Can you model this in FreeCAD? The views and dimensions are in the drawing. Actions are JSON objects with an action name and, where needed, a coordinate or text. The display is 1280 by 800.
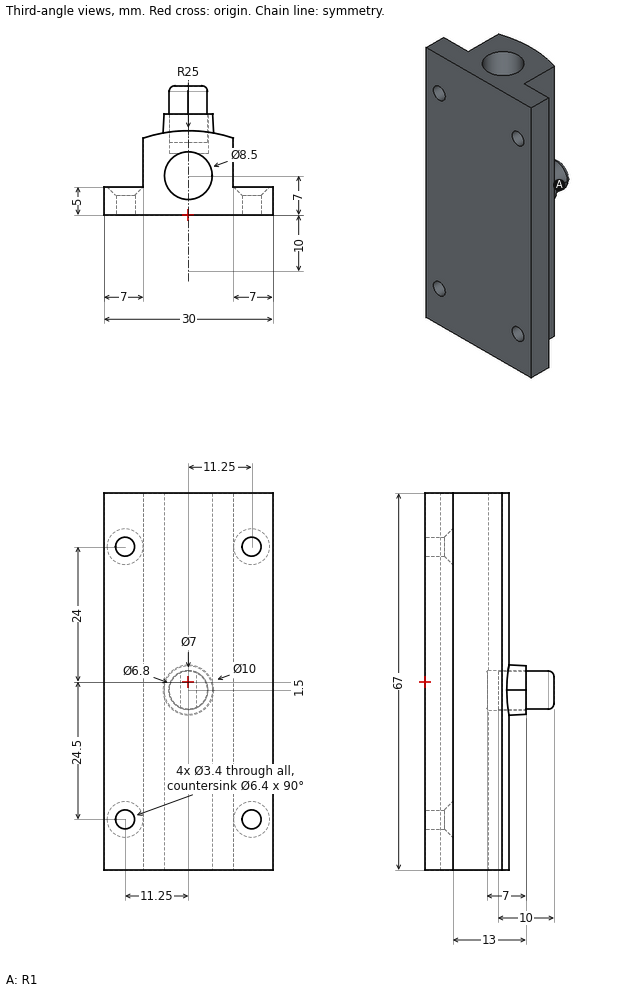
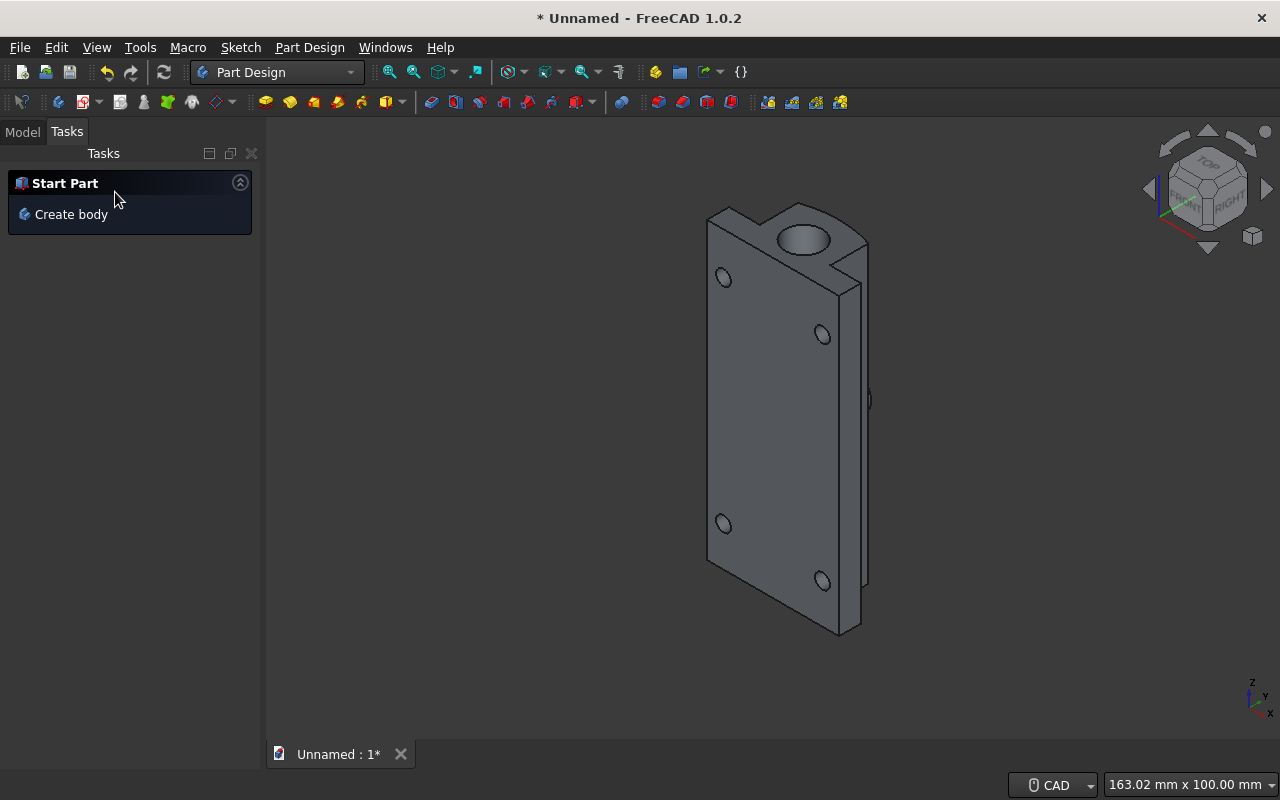
{"action": "left_click", "coordinate": [60, 102]}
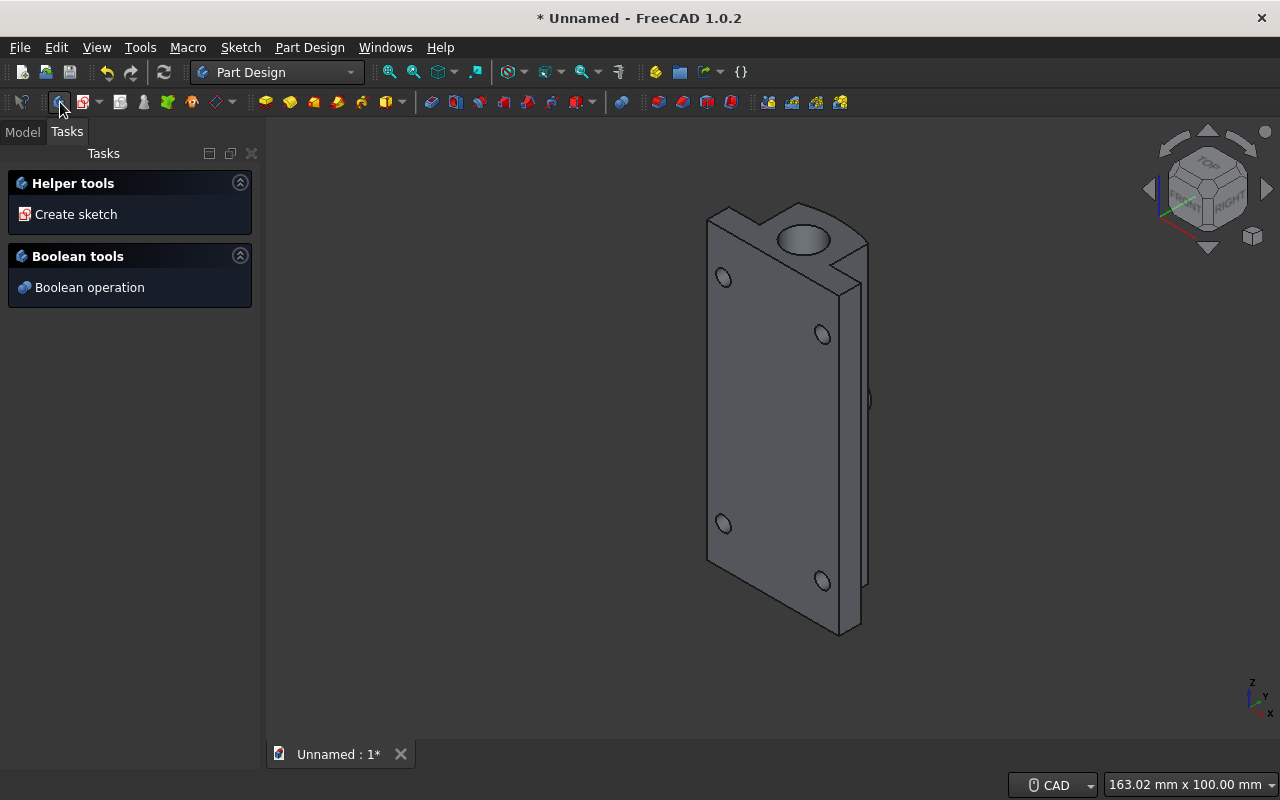
{"action": "left_click", "coordinate": [23, 131]}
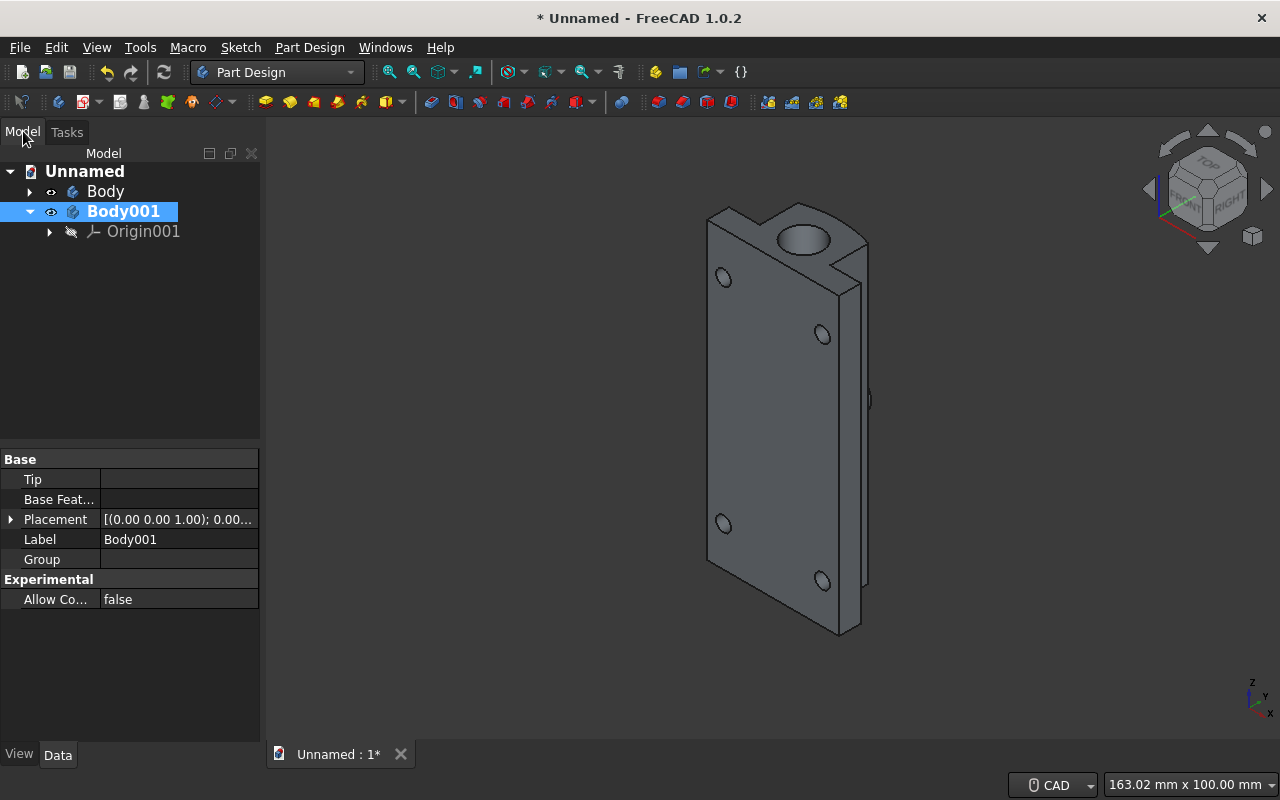
{"action": "left_click", "coordinate": [50, 232]}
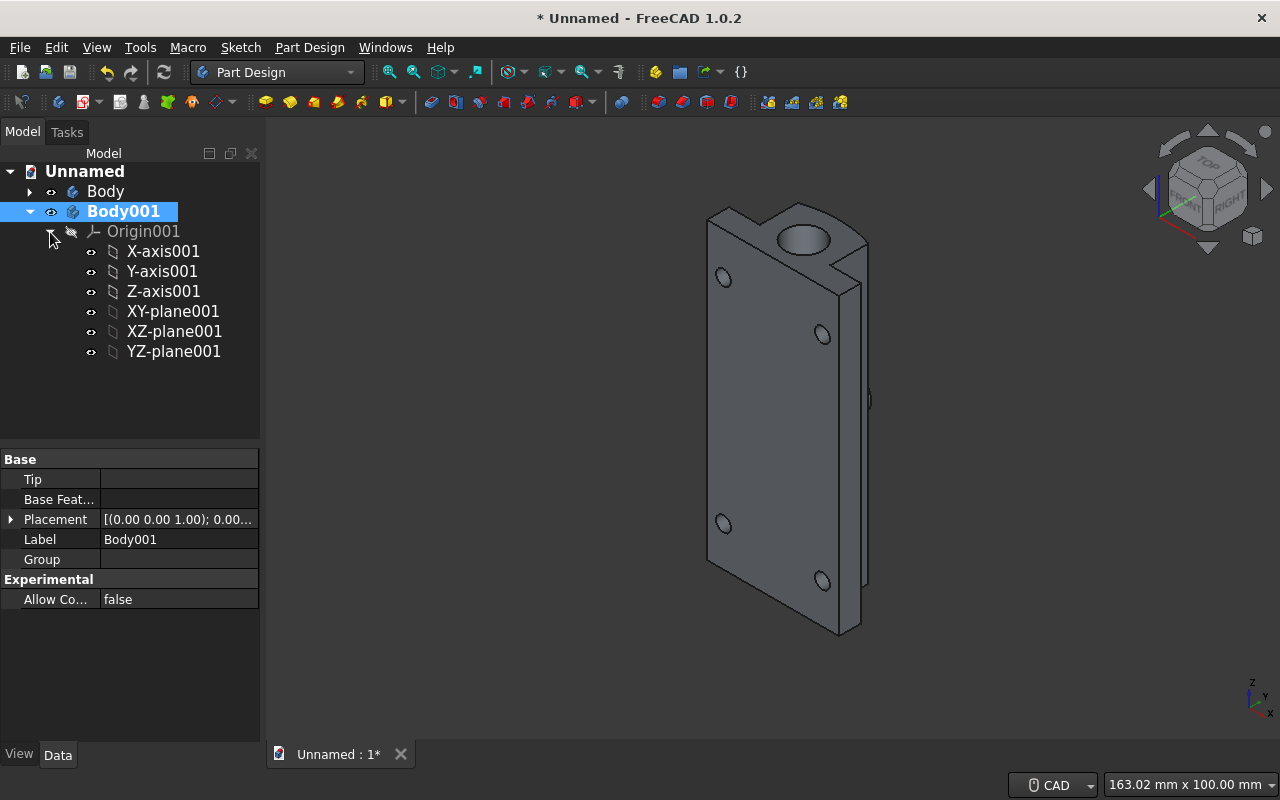
{"action": "left_click", "coordinate": [136, 332]}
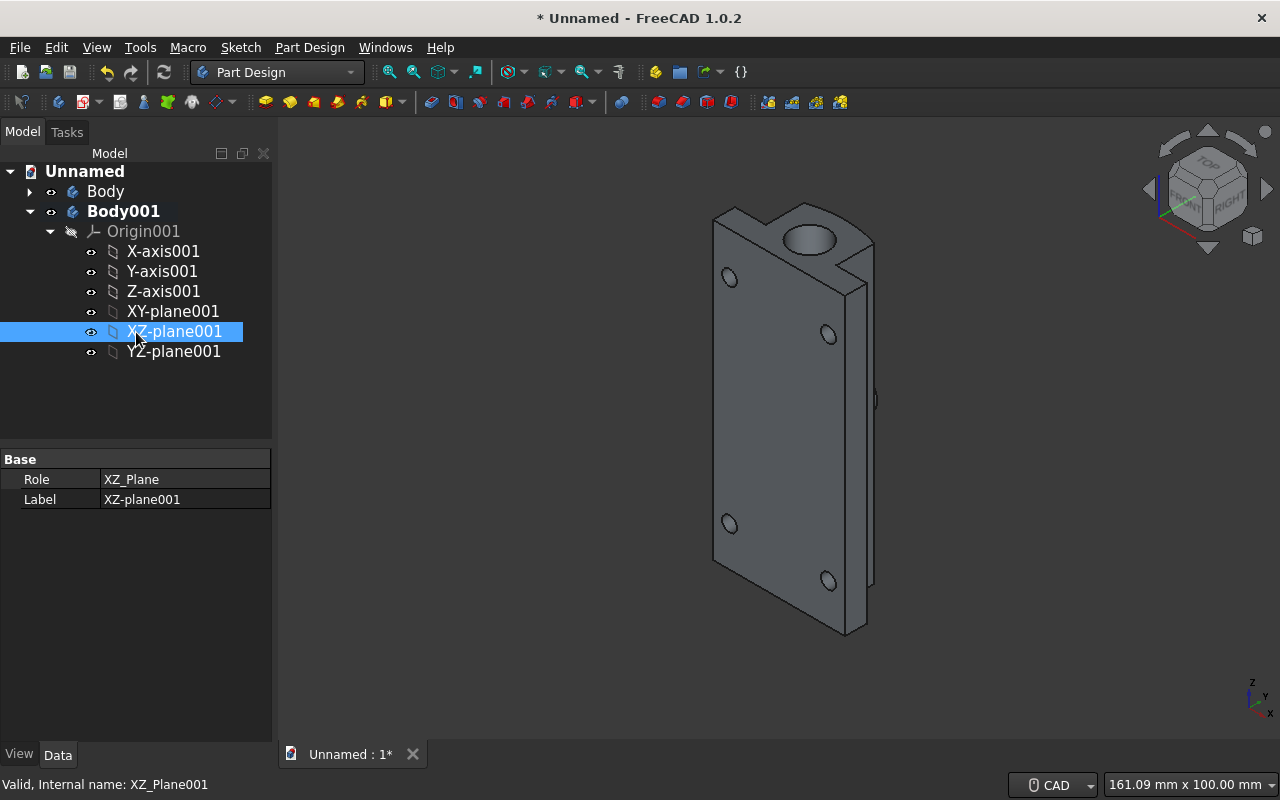
{"action": "left_click", "coordinate": [216, 102]}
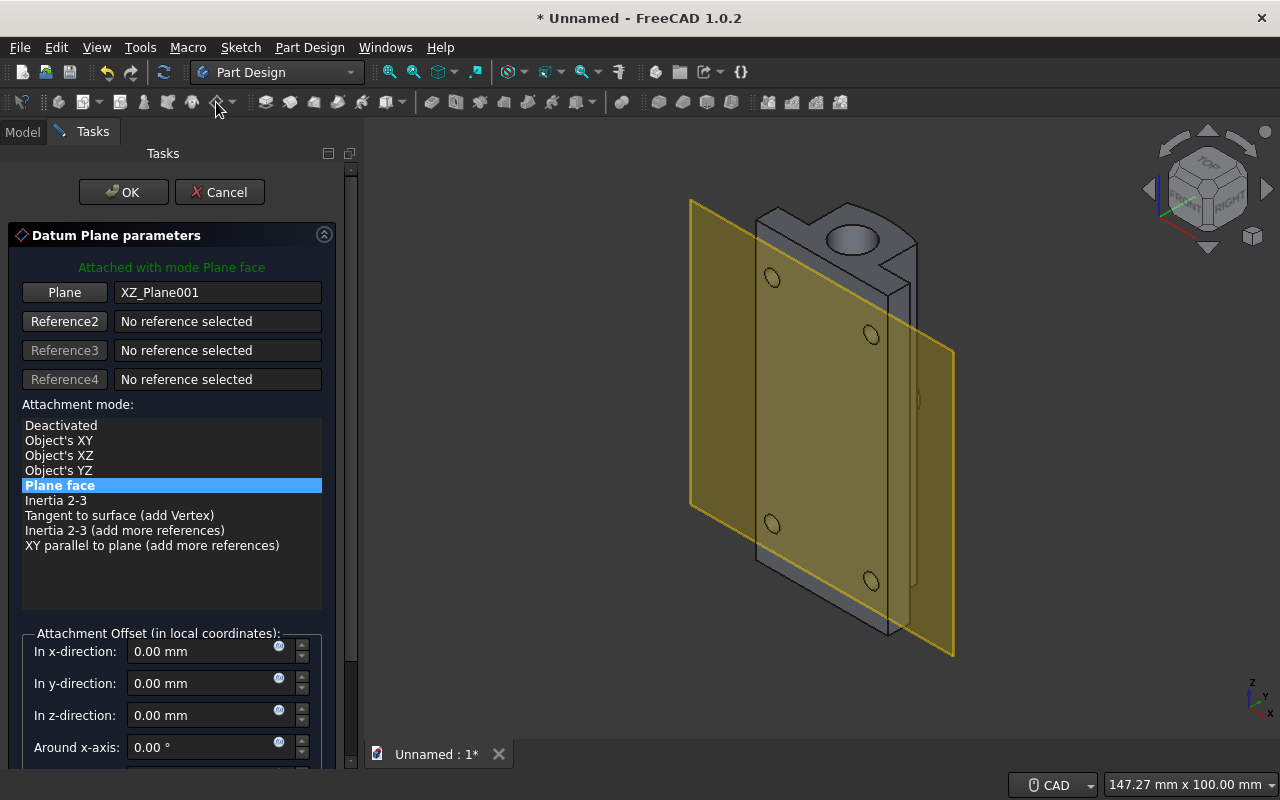
{"action": "triple_click", "coordinate": [210, 715]}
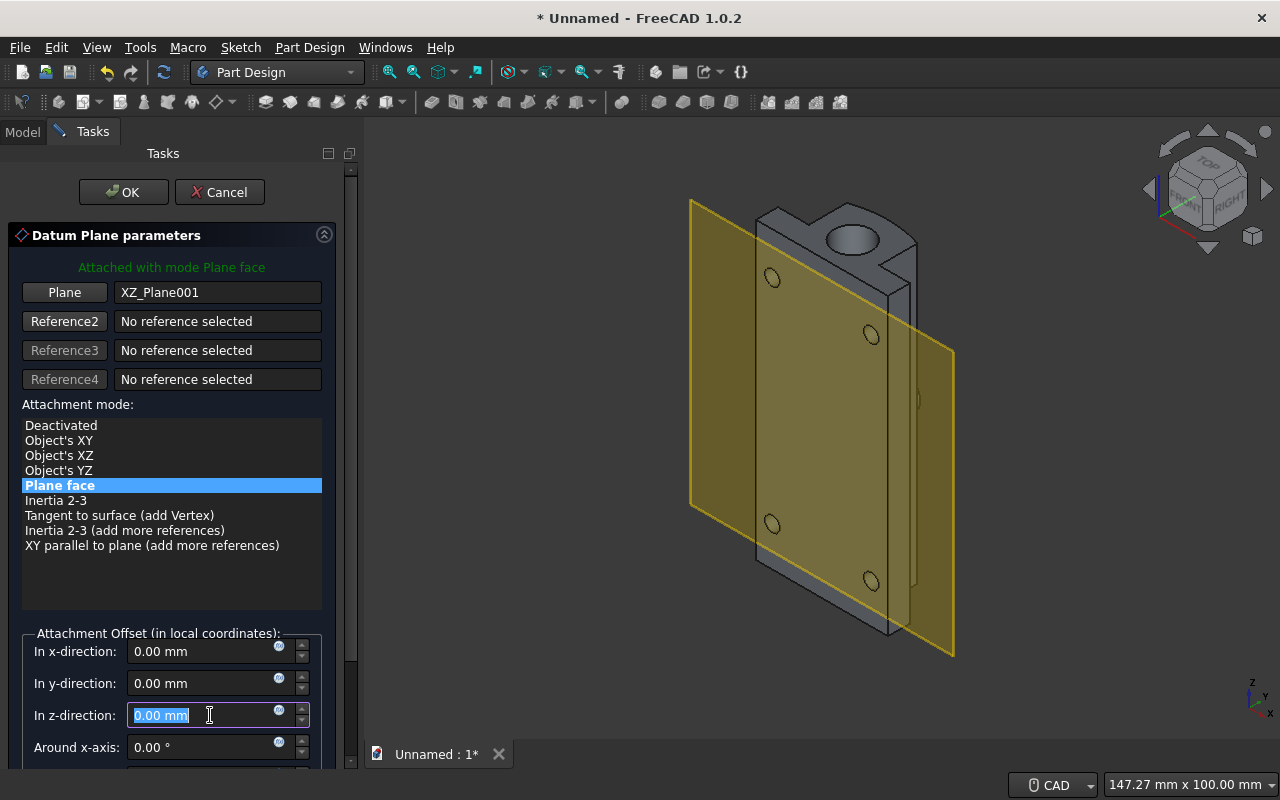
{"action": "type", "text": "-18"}
{"action": "key", "text": "Tab"}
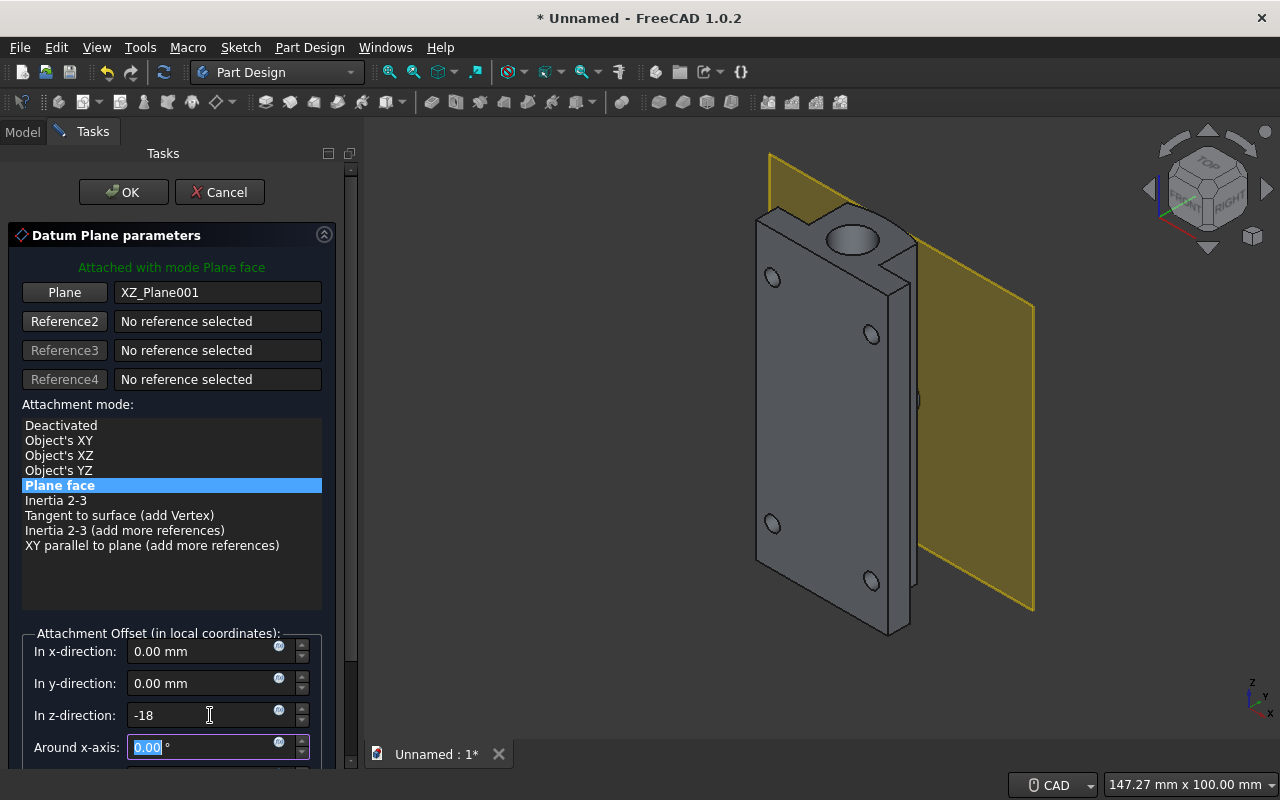
{"action": "left_click", "coordinate": [124, 192]}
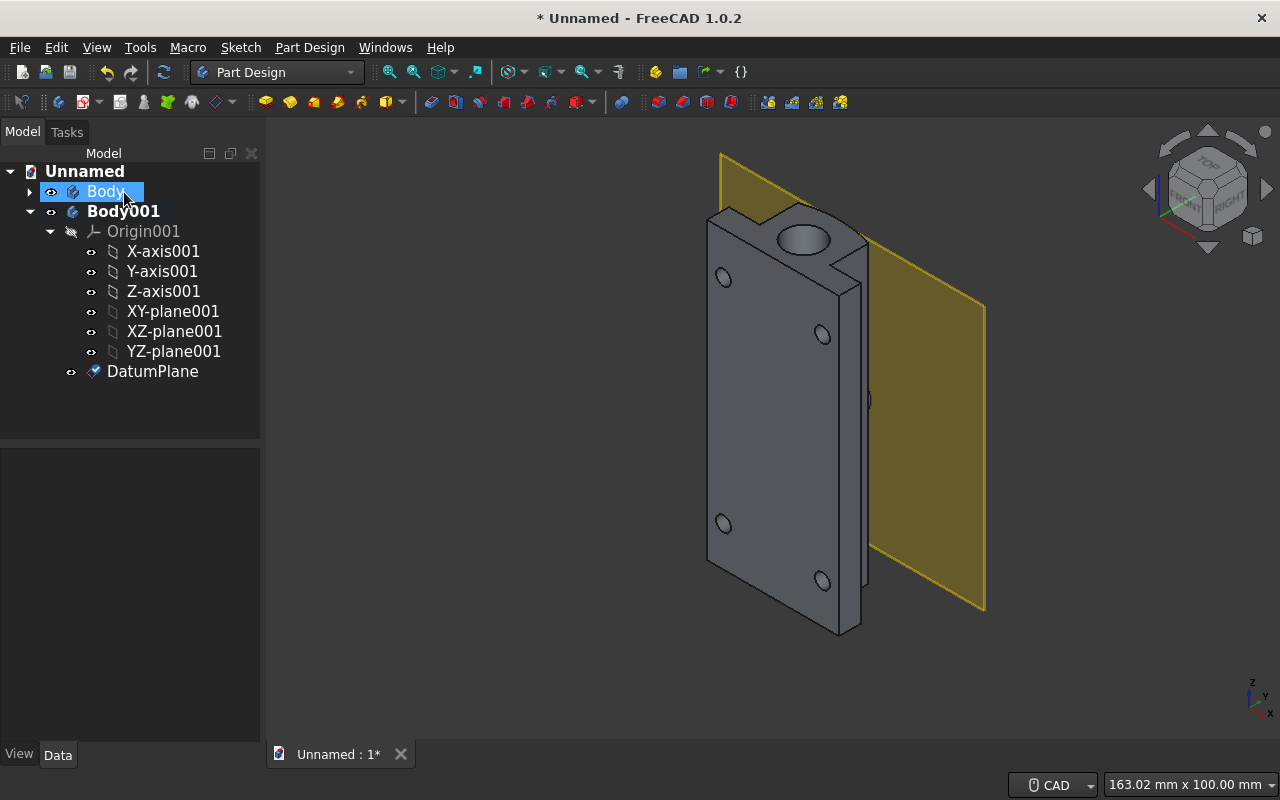
{"action": "left_click", "coordinate": [116, 372]}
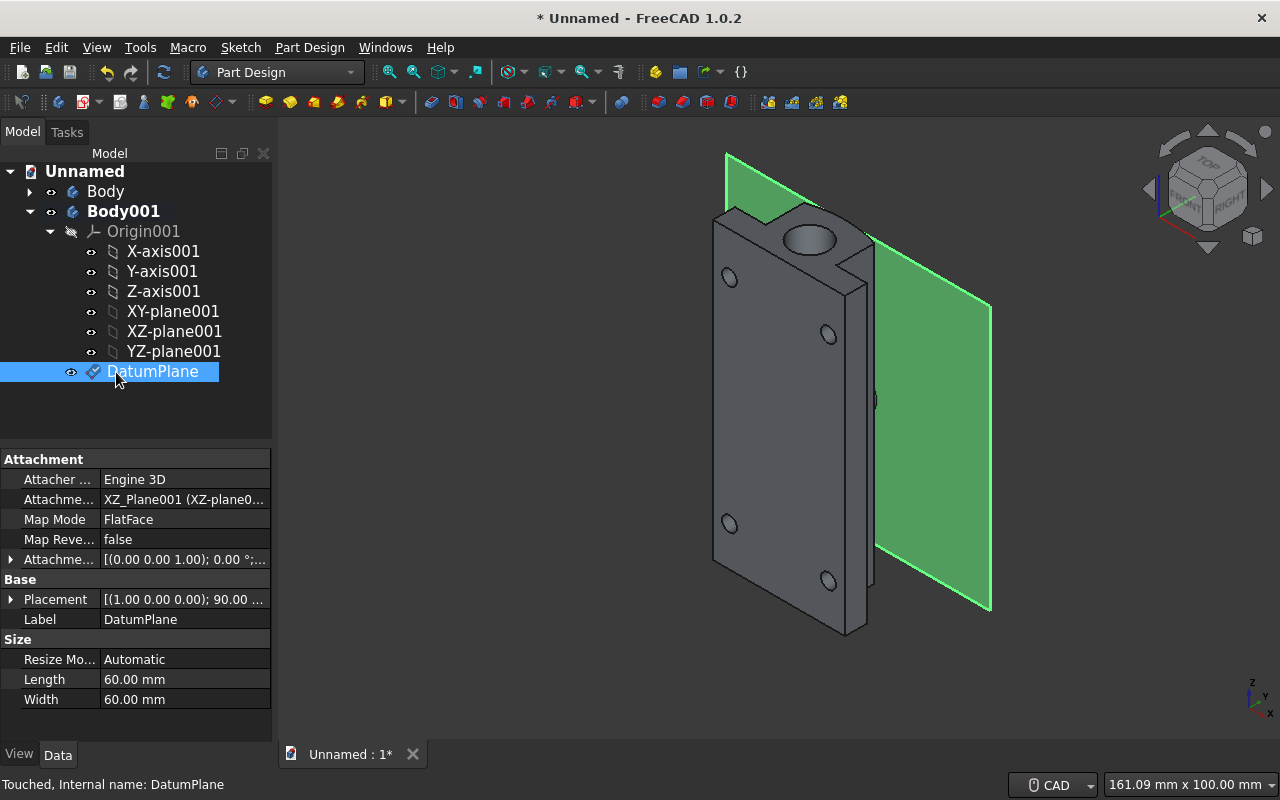
{"action": "left_click", "coordinate": [84, 102]}